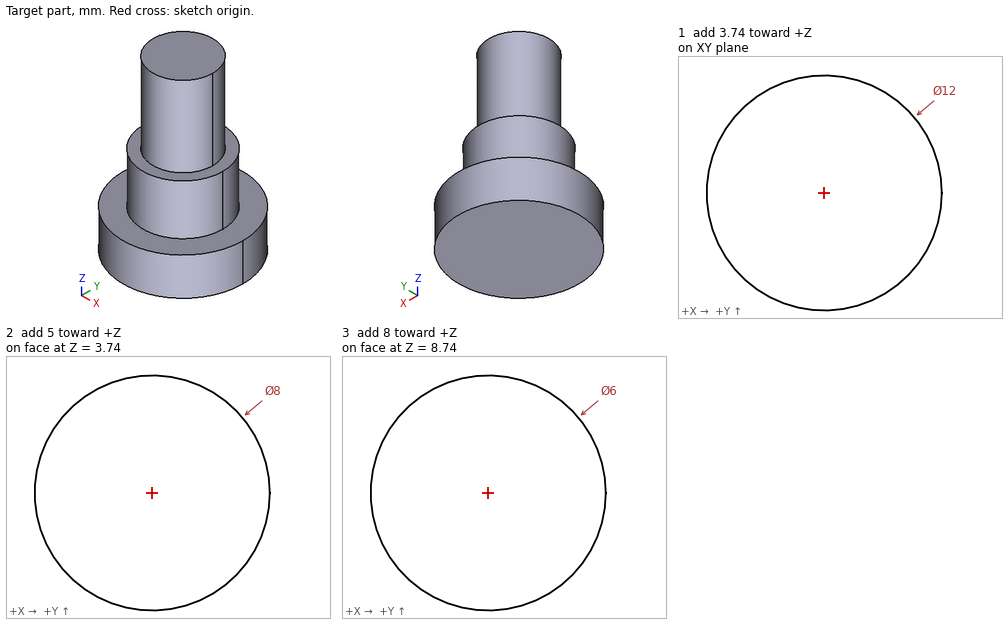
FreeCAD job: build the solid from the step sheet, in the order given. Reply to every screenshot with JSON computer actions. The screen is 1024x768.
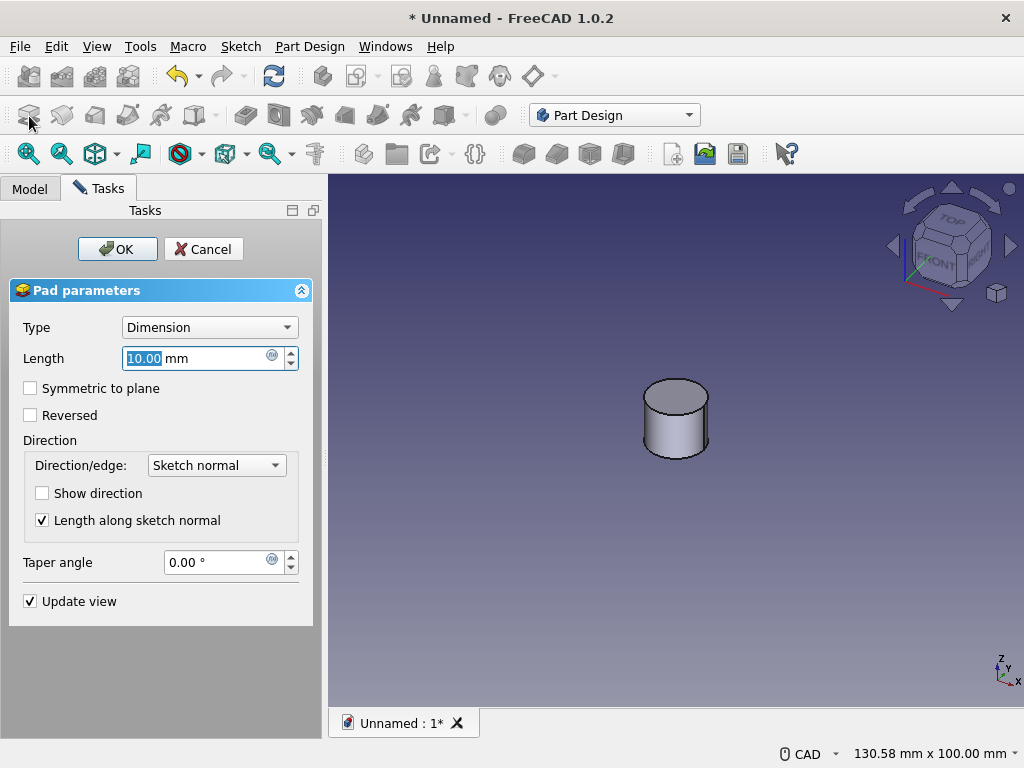
{"action": "type", "text": "3.74"}
{"action": "key", "text": "Tab"}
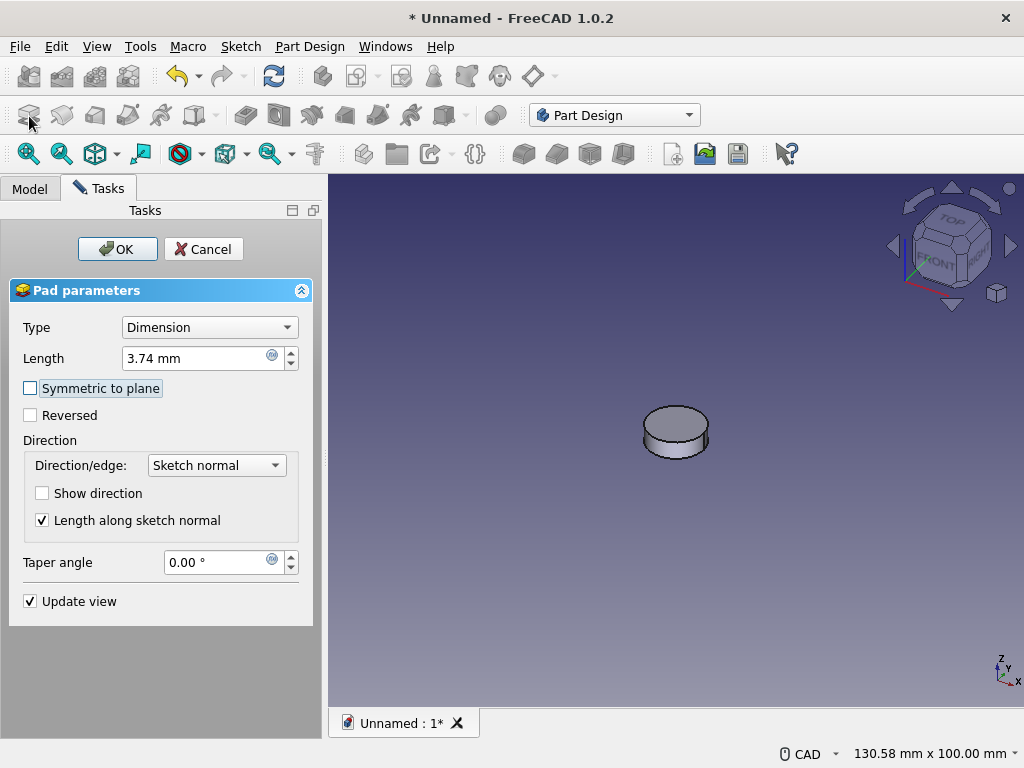
{"action": "left_click", "coordinate": [118, 249]}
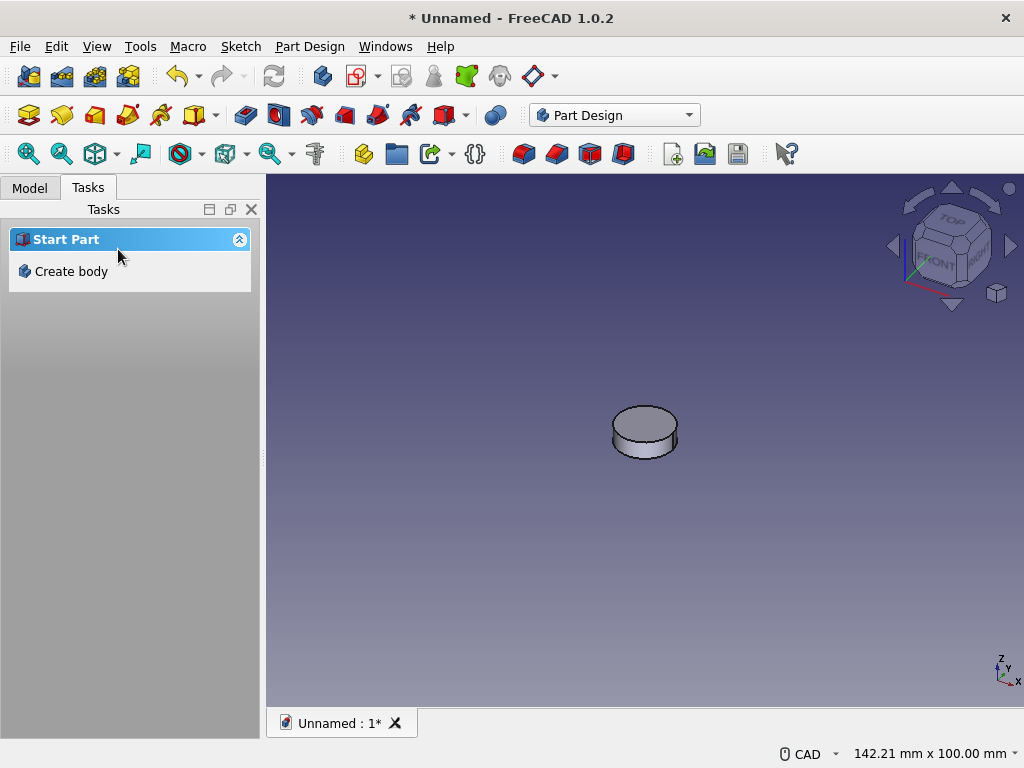
{"action": "left_click", "coordinate": [29, 154]}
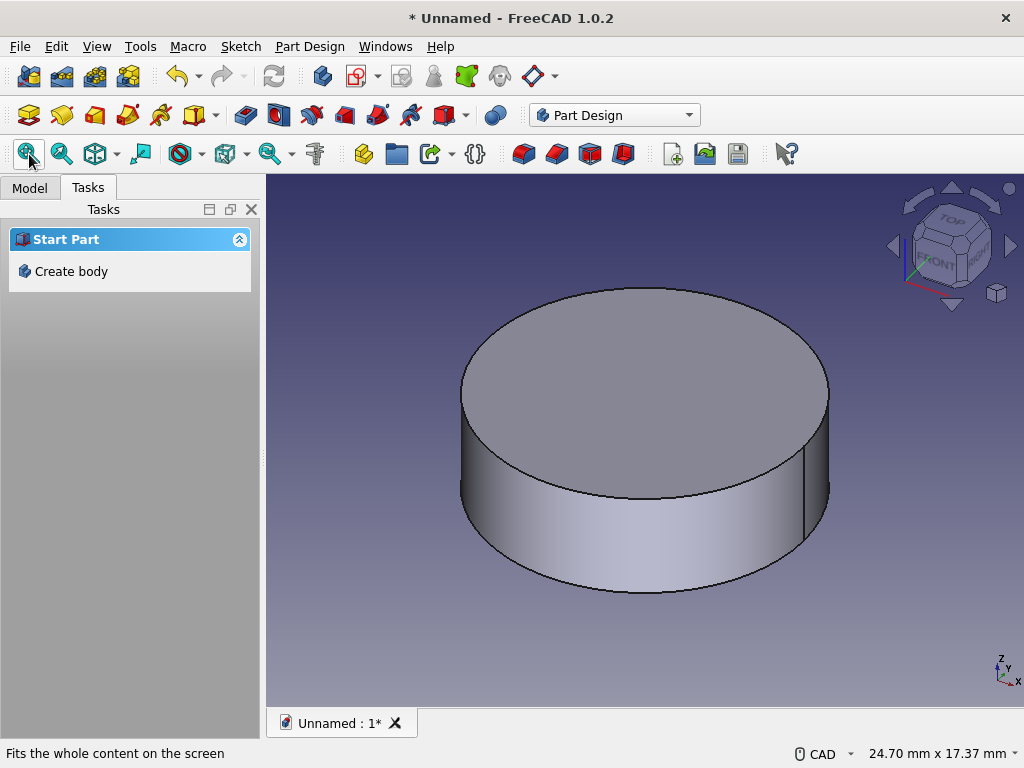
{"action": "left_click", "coordinate": [645, 392]}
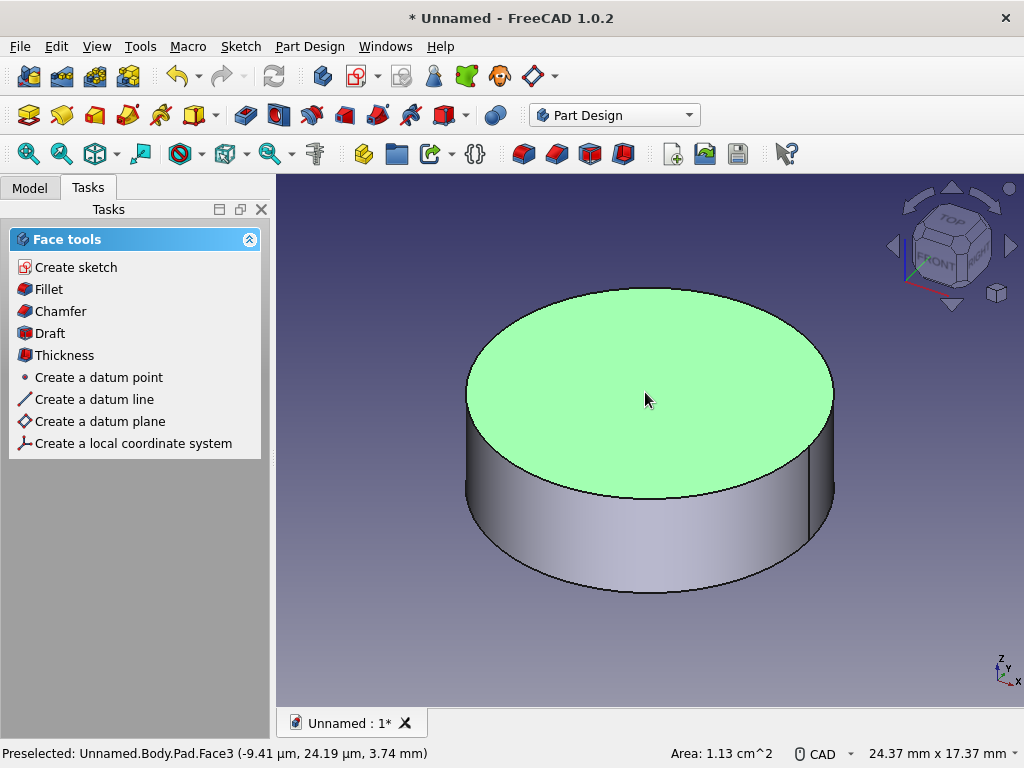
{"action": "left_click", "coordinate": [356, 76]}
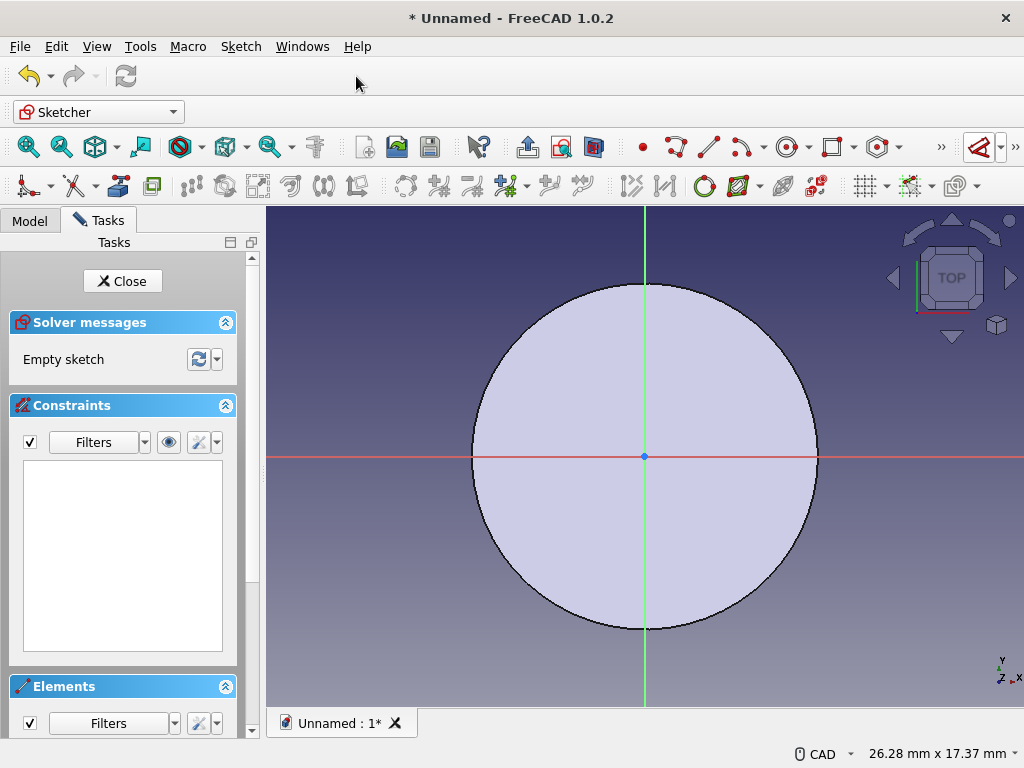
{"action": "scroll", "coordinate": [784, 456], "scroll_direction": "up", "scroll_amount": 2}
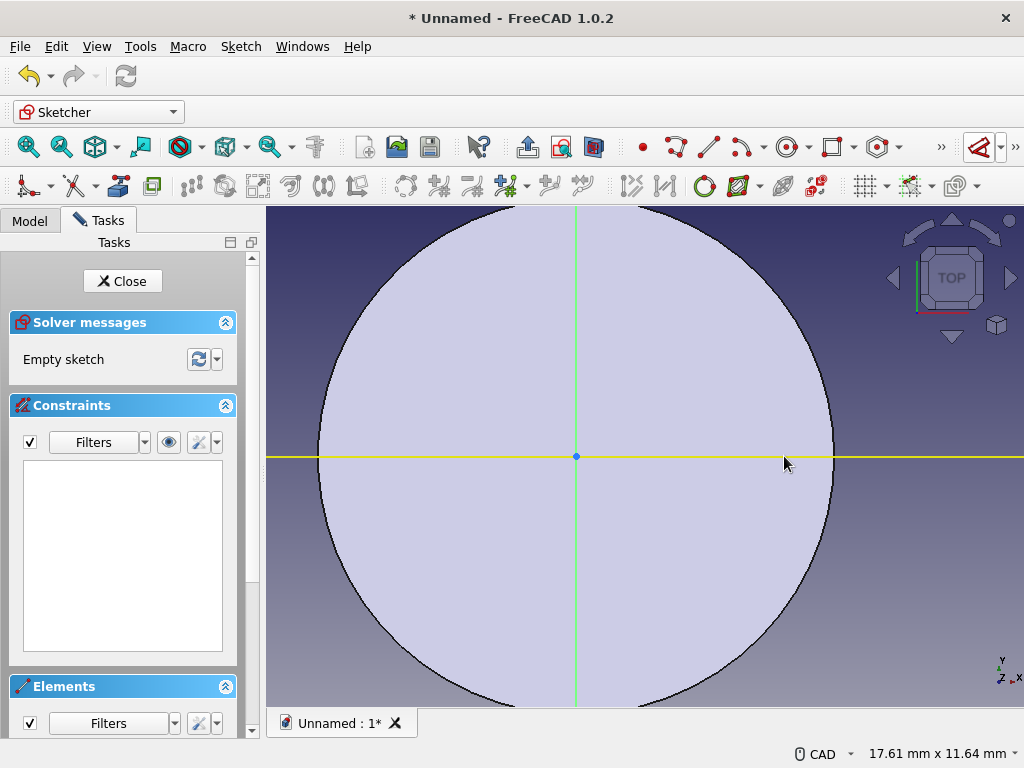
{"action": "left_click", "coordinate": [786, 148]}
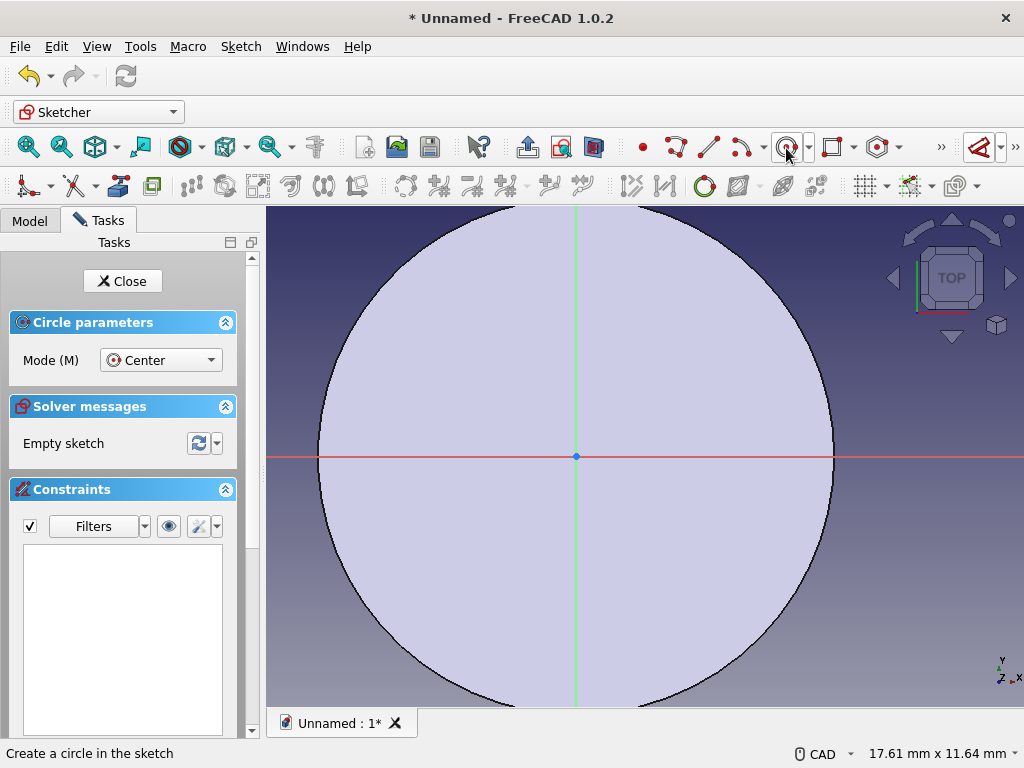
{"action": "left_click", "coordinate": [576, 456]}
{"action": "left_click", "coordinate": [698, 335]}
{"action": "key", "text": "Escape"}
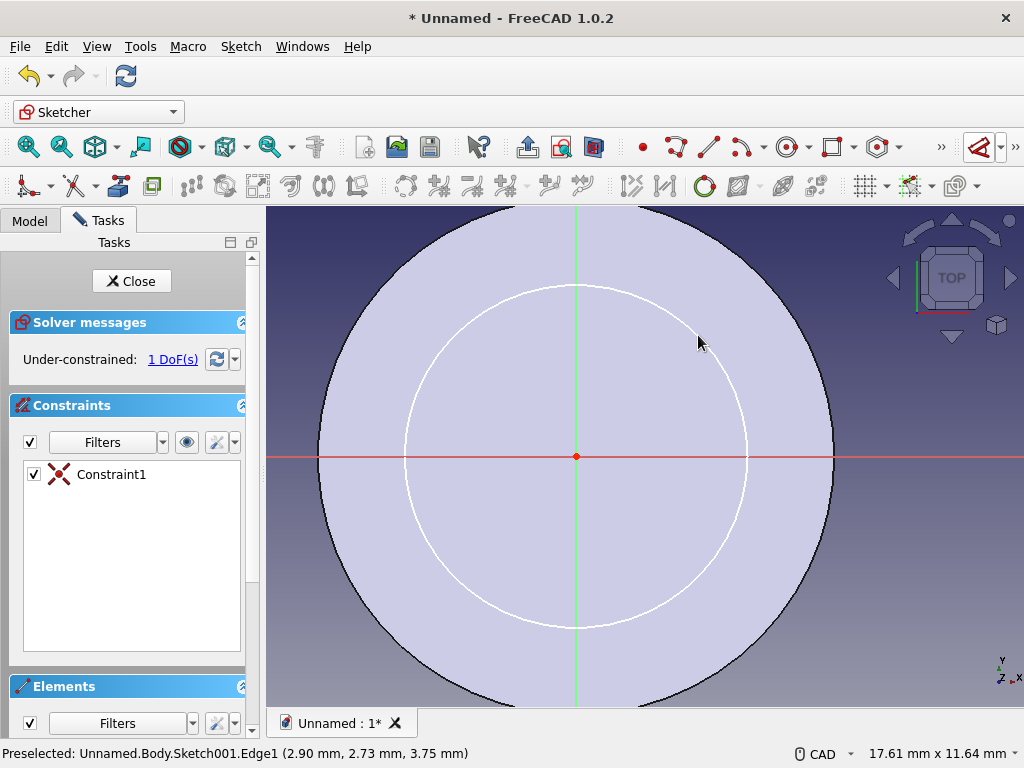
{"action": "left_click", "coordinate": [697, 335]}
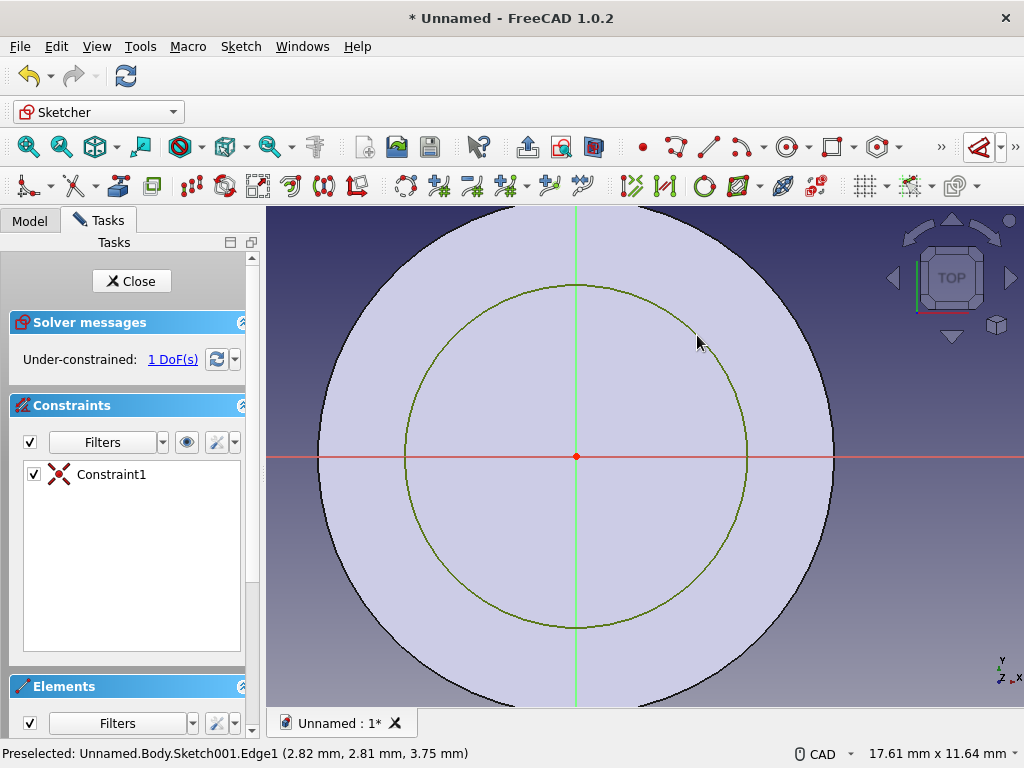
{"action": "left_click", "coordinate": [1000, 148]}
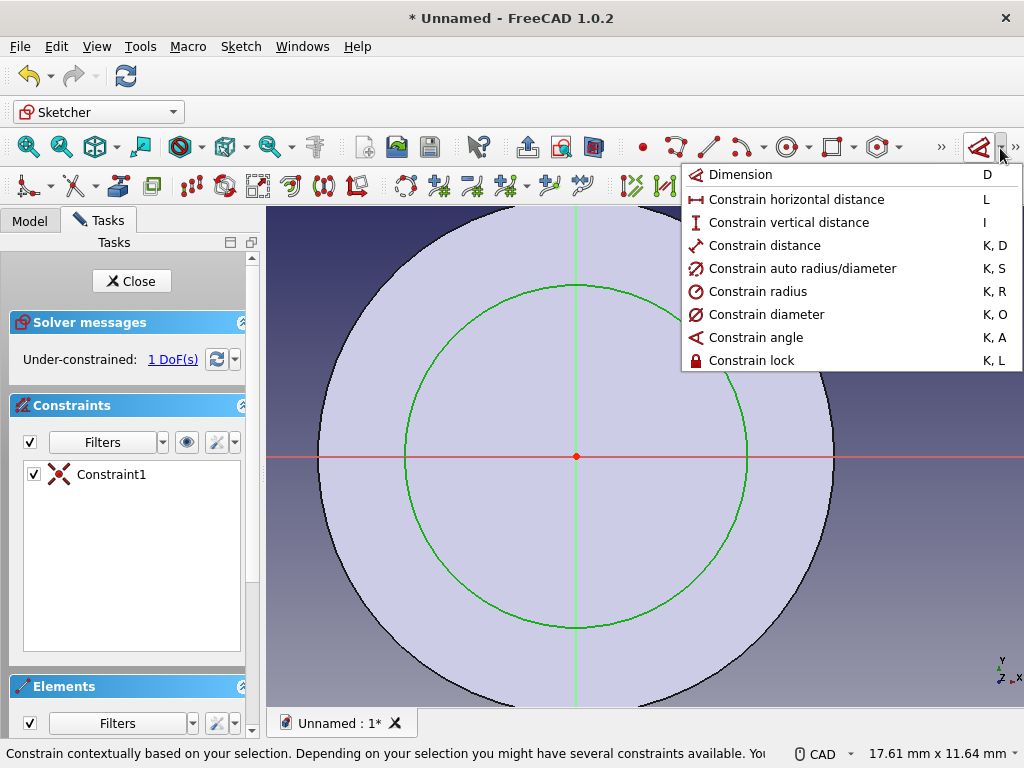
{"action": "left_click", "coordinate": [852, 314]}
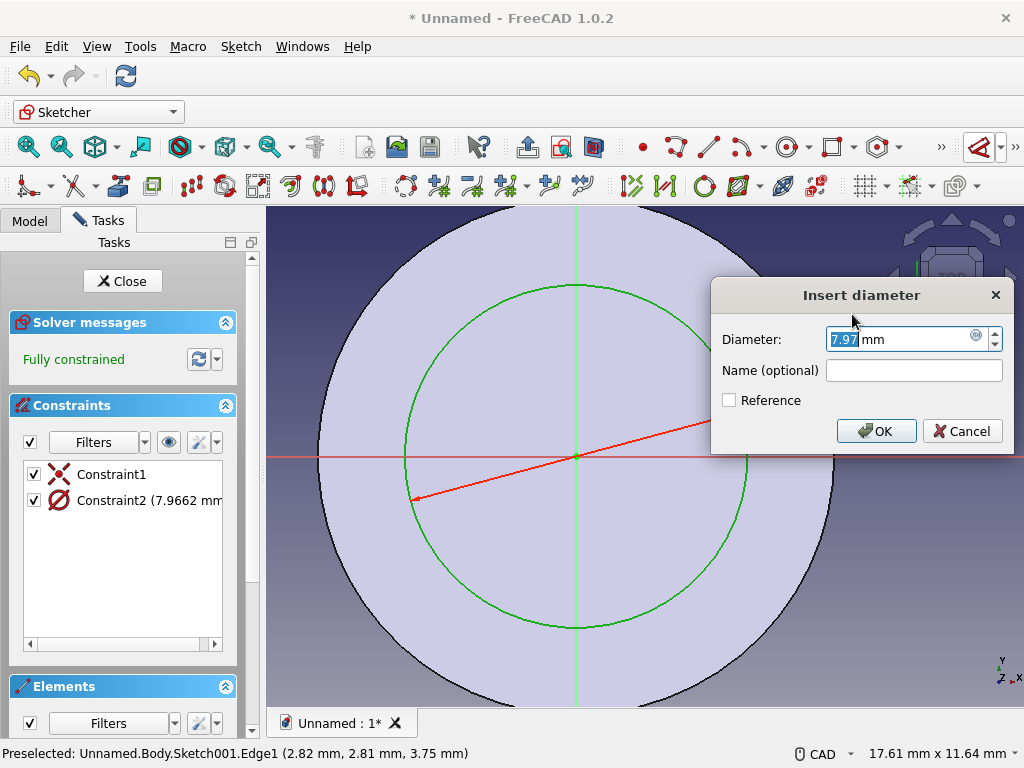
{"action": "type", "text": "8"}
{"action": "key", "text": "Return"}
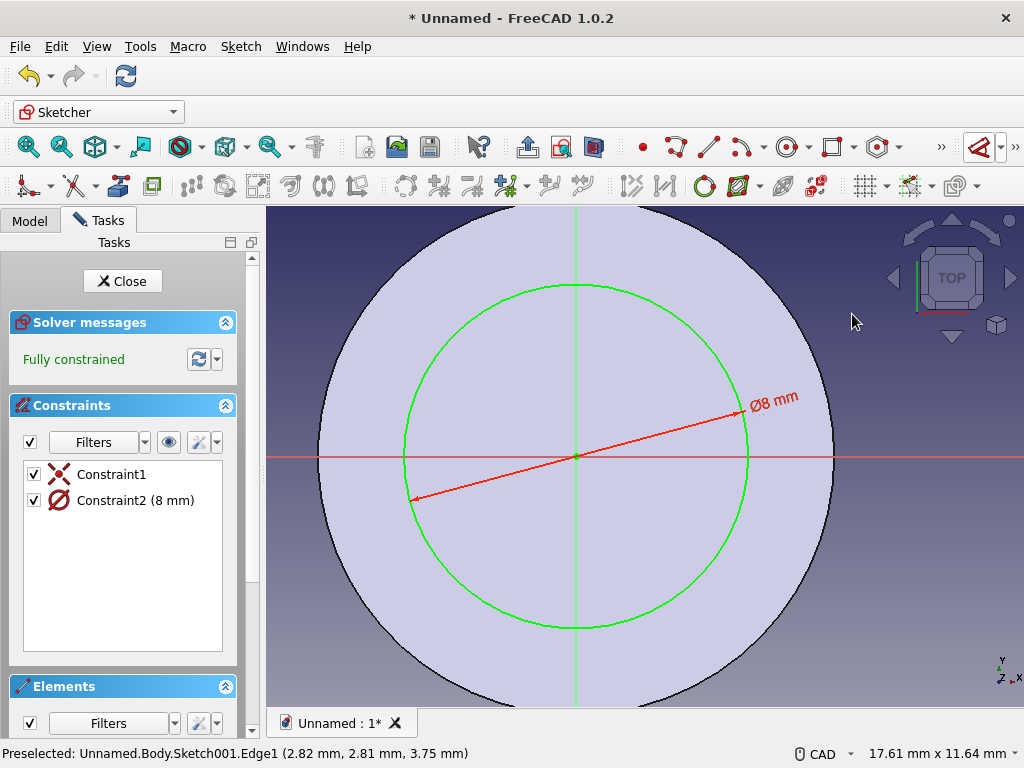
{"action": "left_click", "coordinate": [123, 281]}